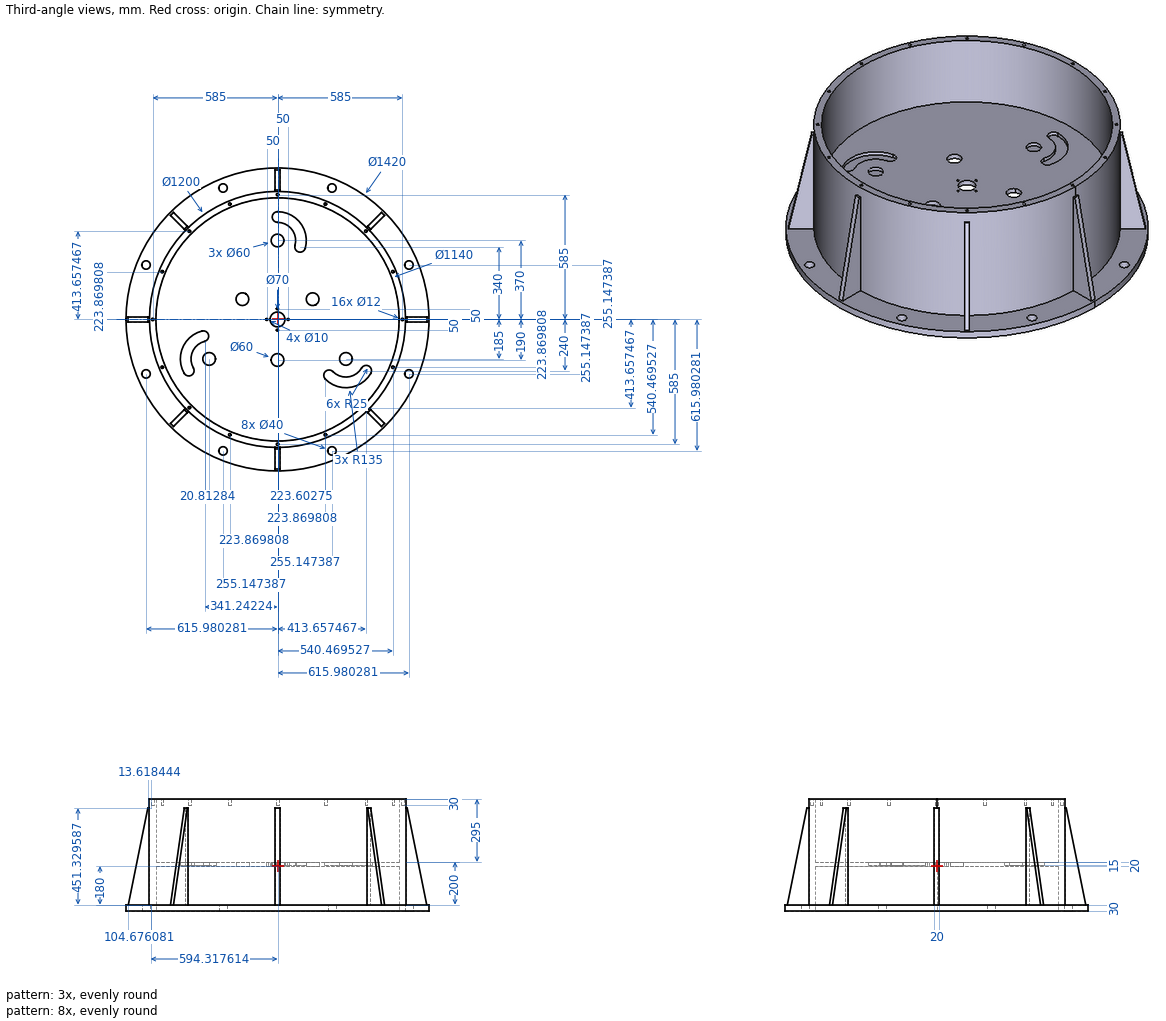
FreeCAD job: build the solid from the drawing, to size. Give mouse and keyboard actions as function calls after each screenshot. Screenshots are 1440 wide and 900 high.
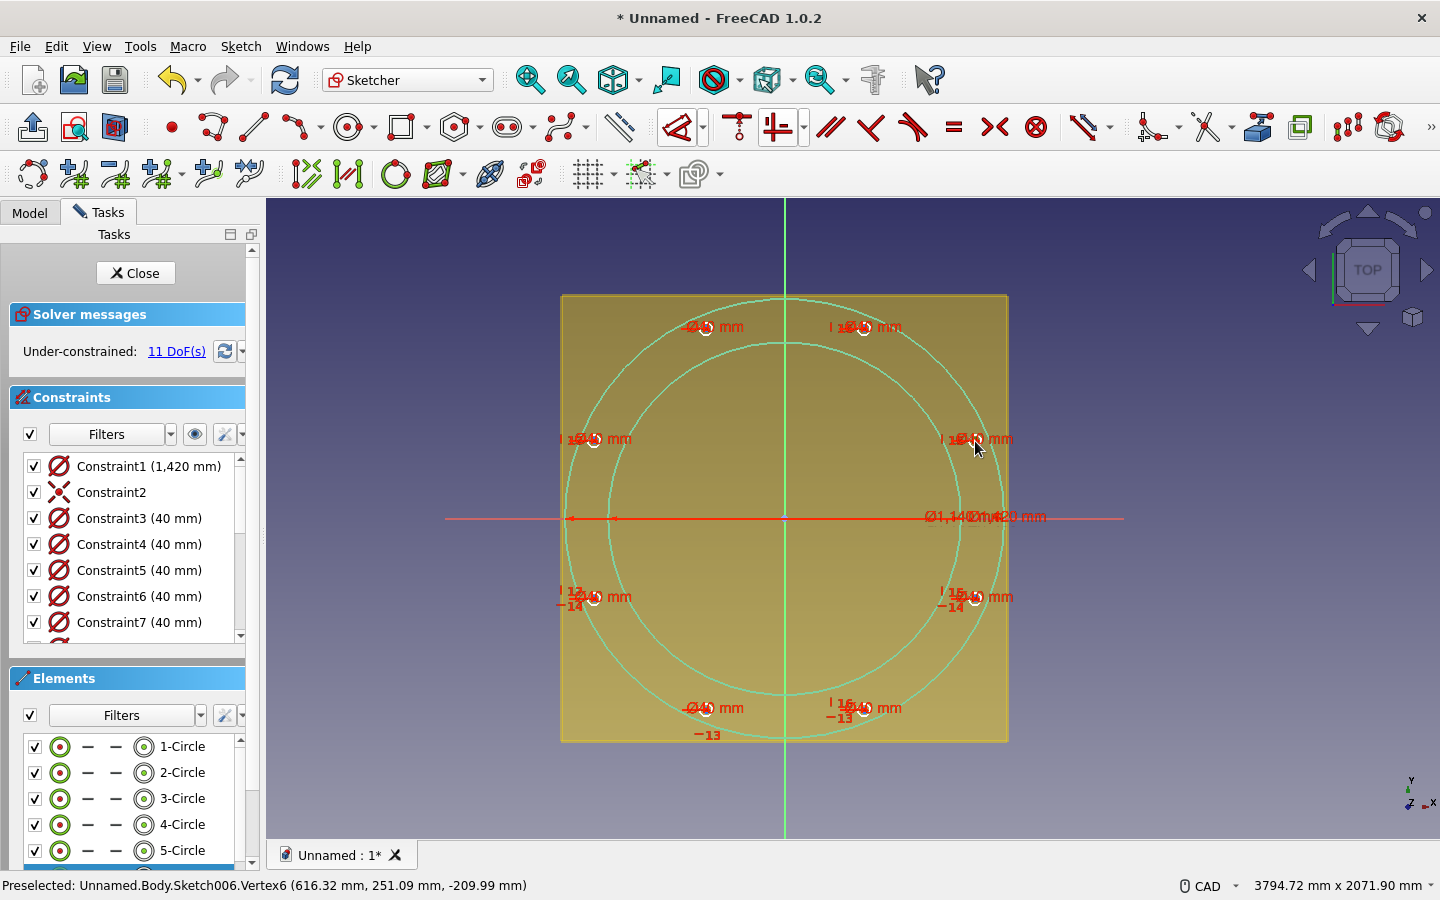
click(594, 441)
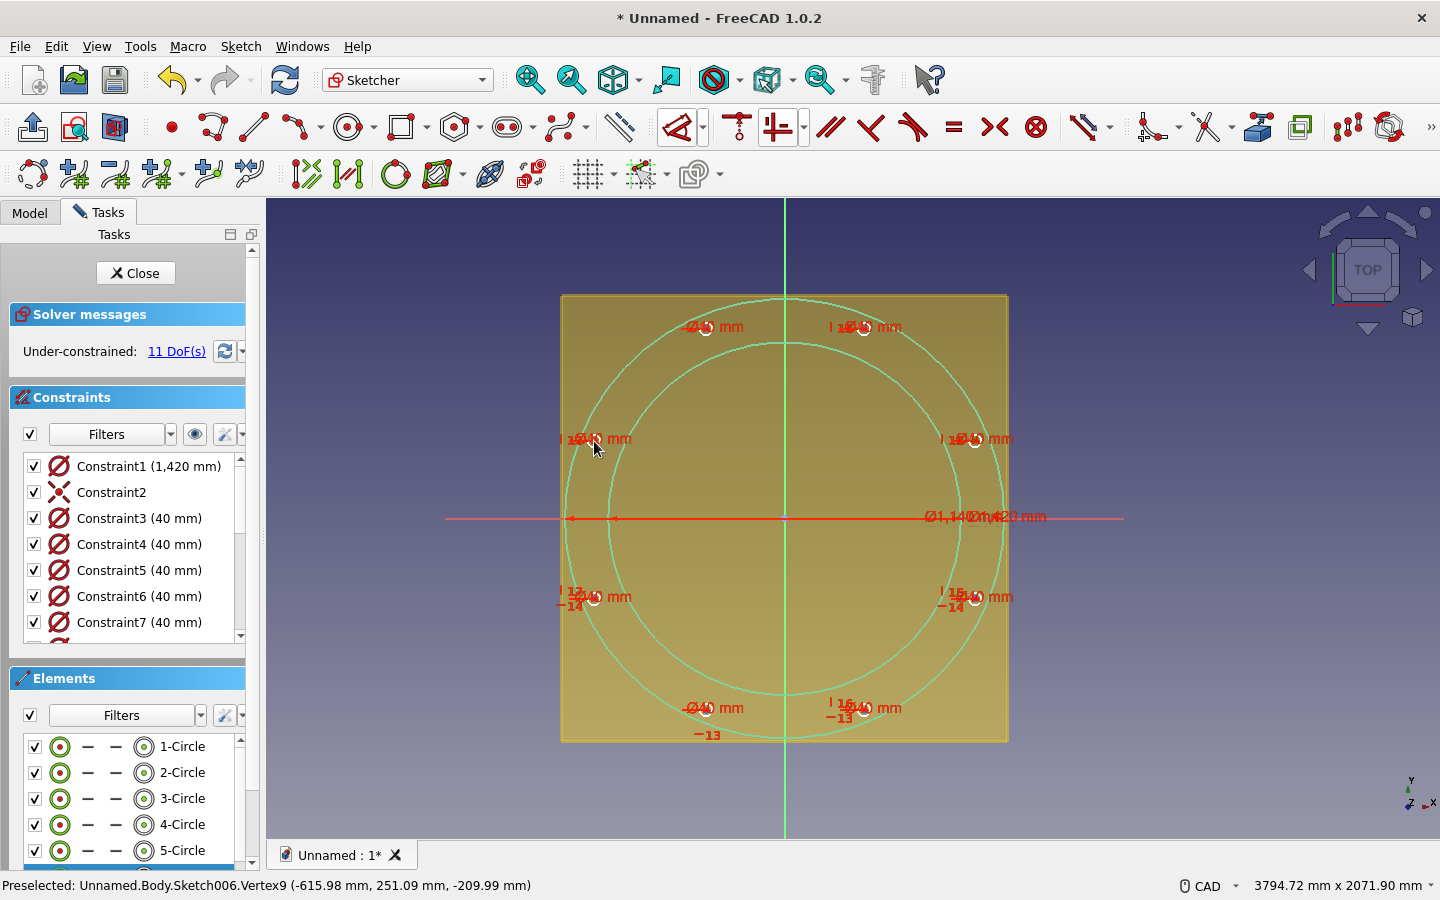
key(h)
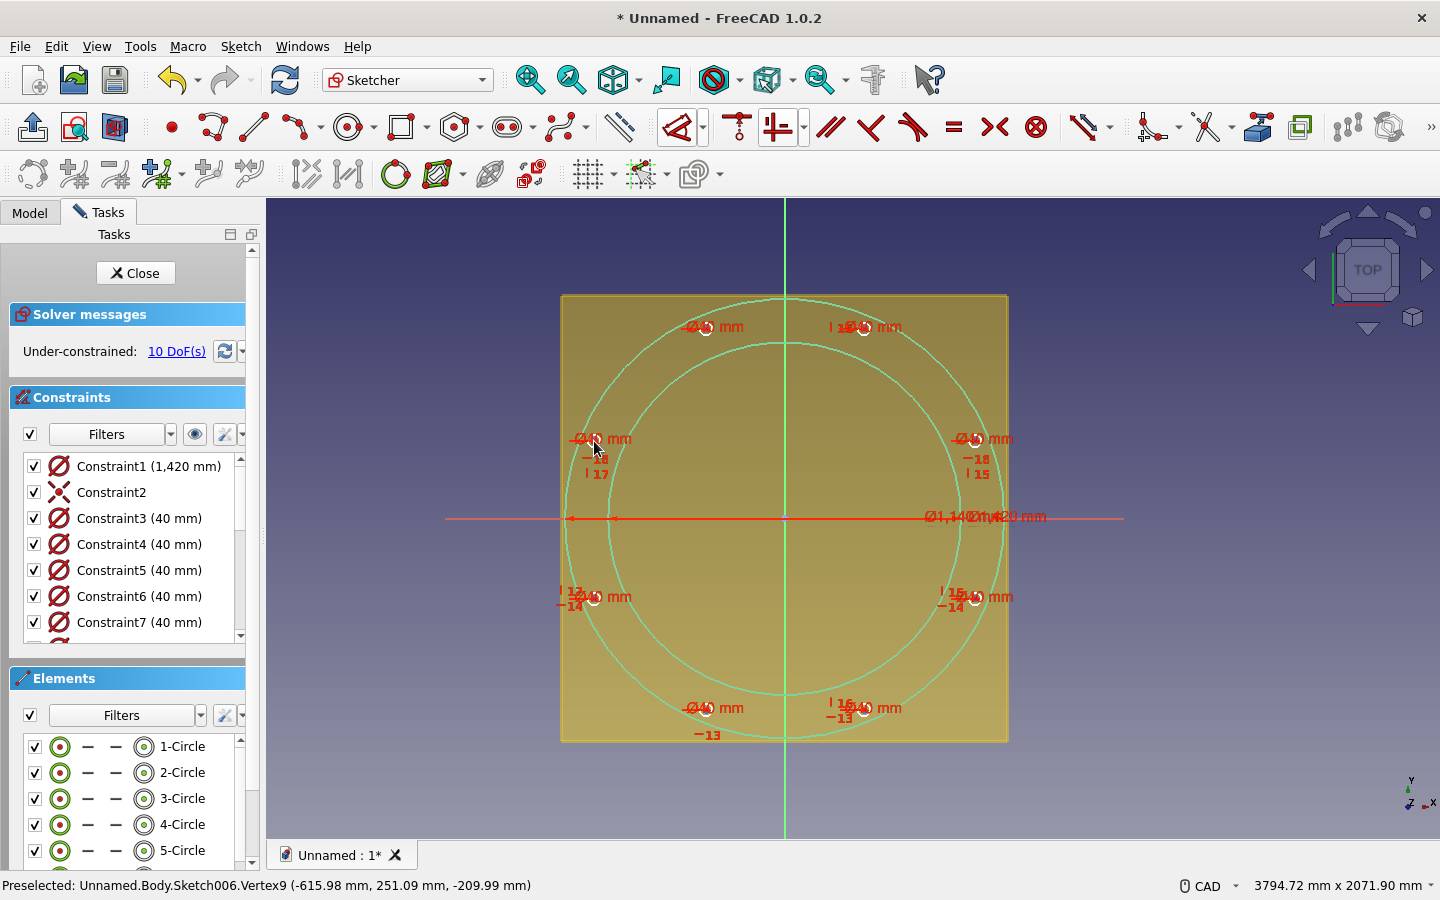
click(864, 329)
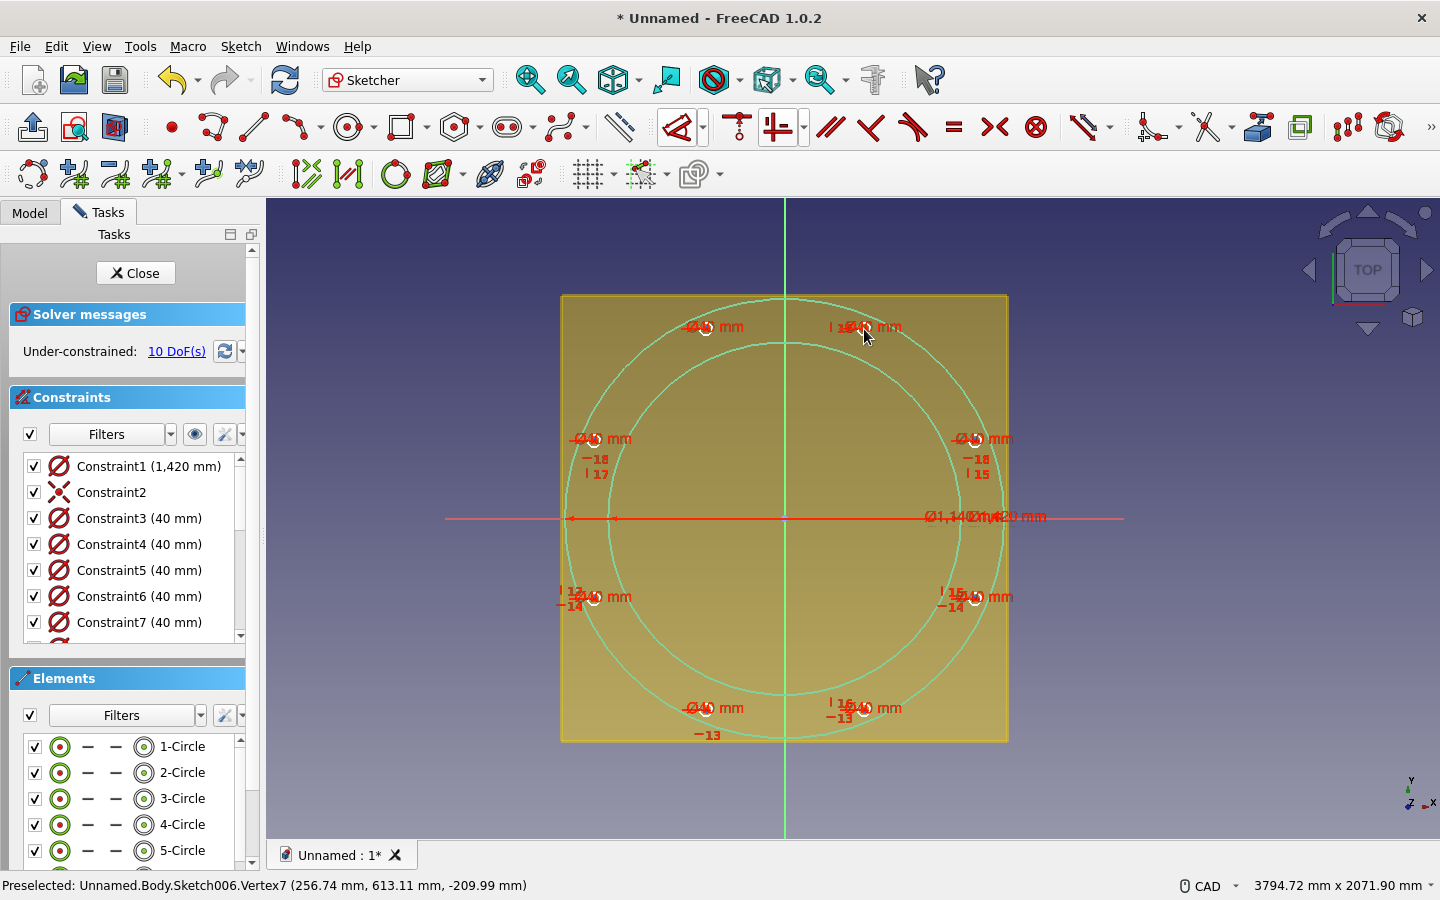
click(706, 329)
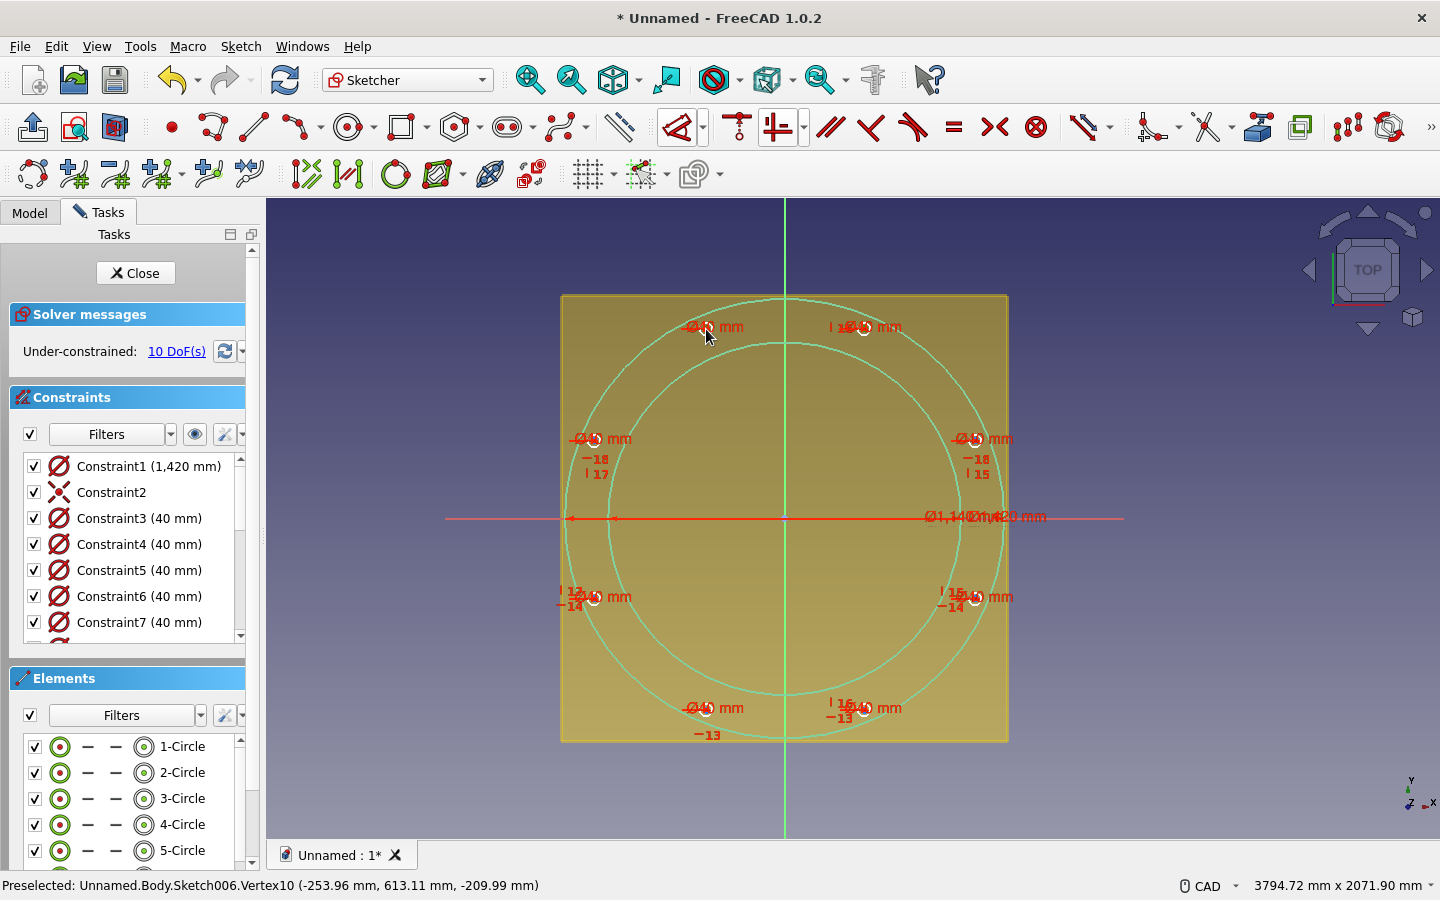
key(h)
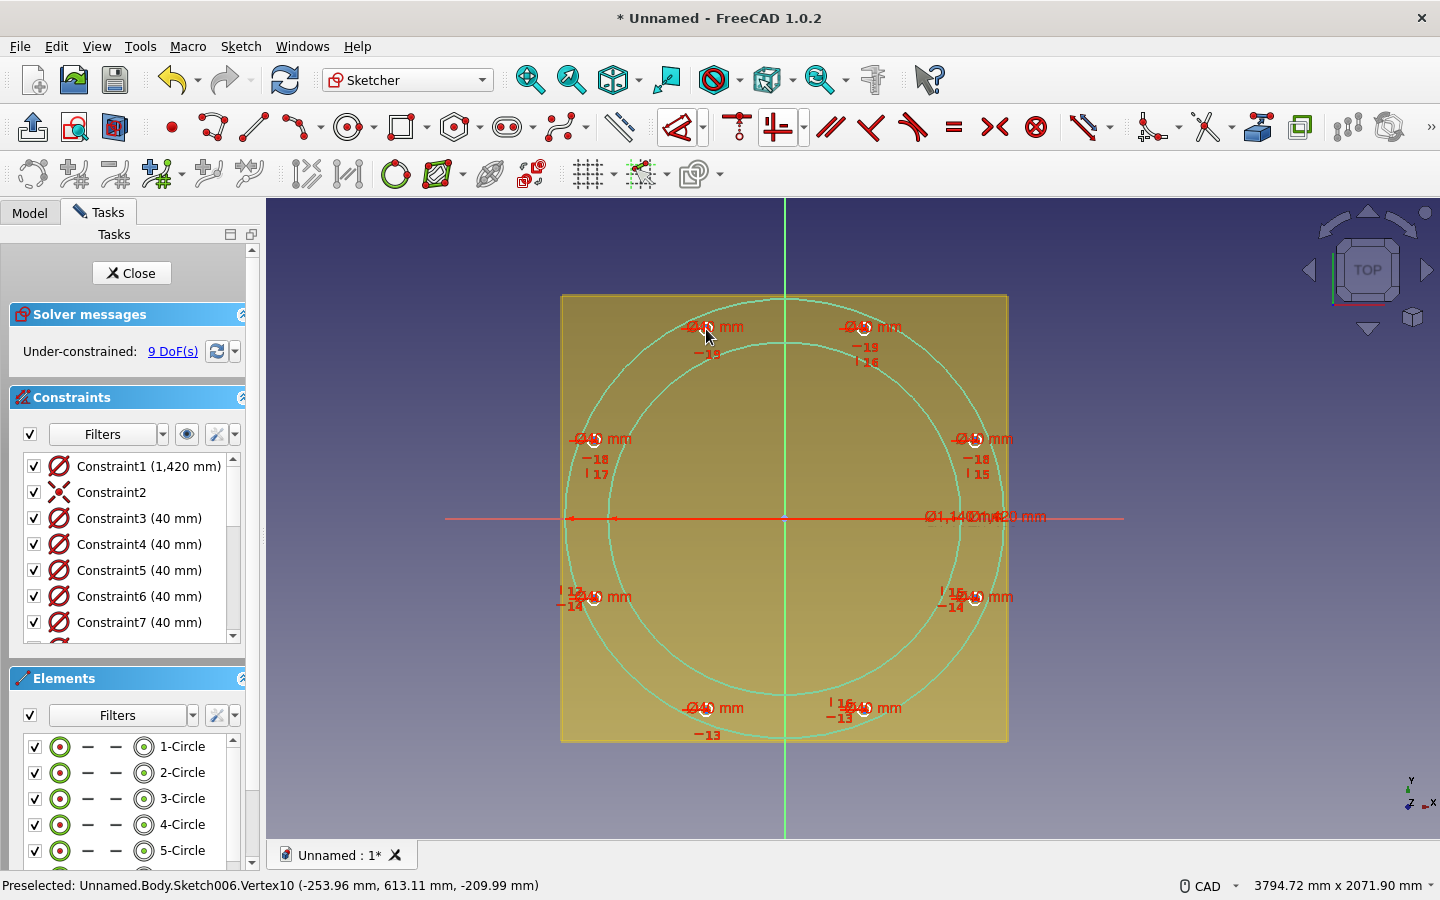
click(706, 710)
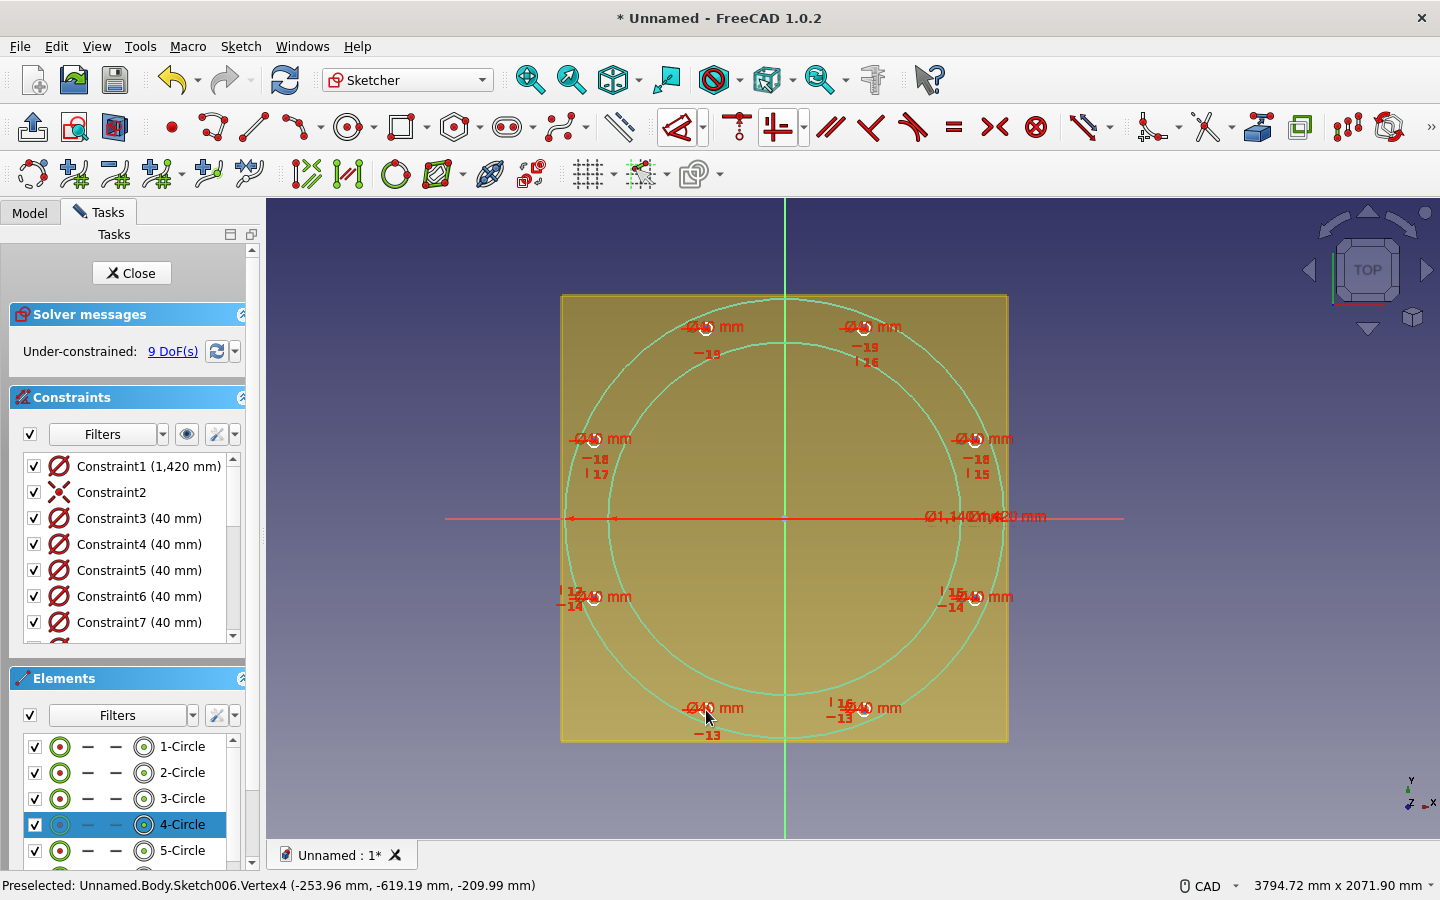
click(706, 329)